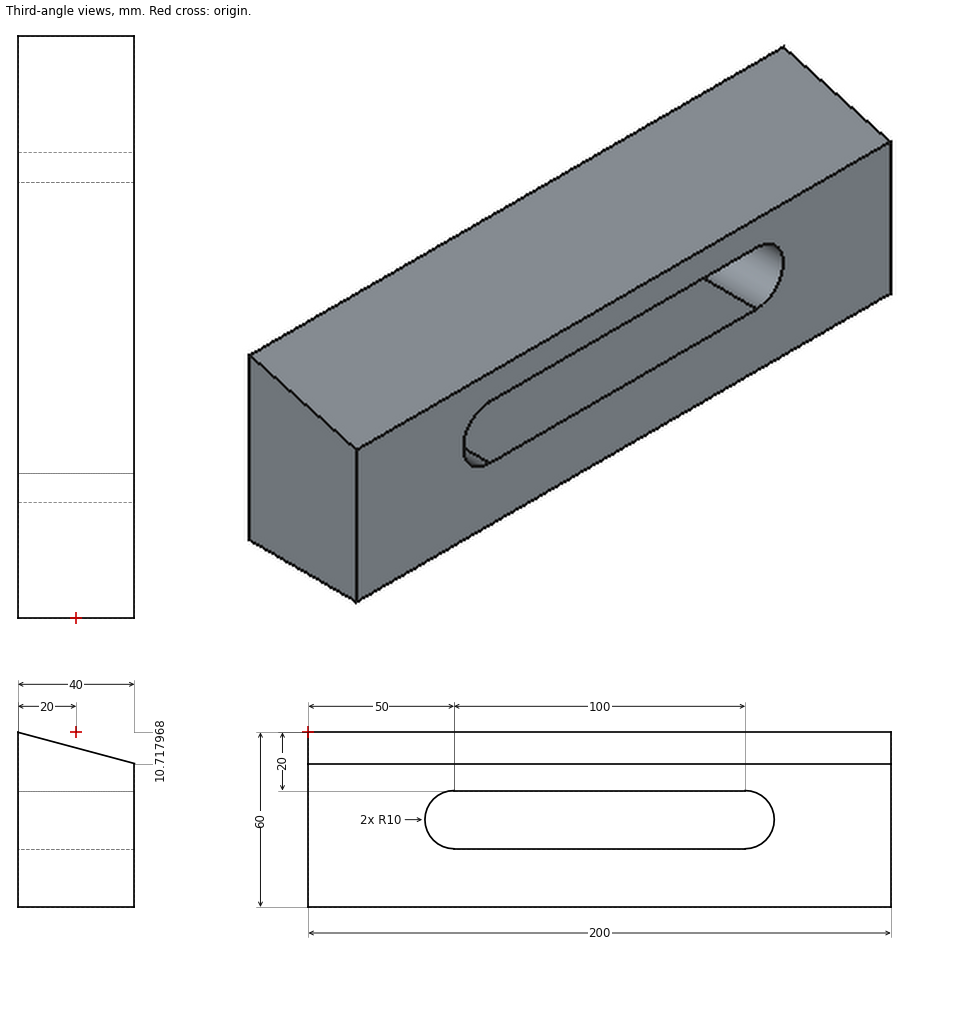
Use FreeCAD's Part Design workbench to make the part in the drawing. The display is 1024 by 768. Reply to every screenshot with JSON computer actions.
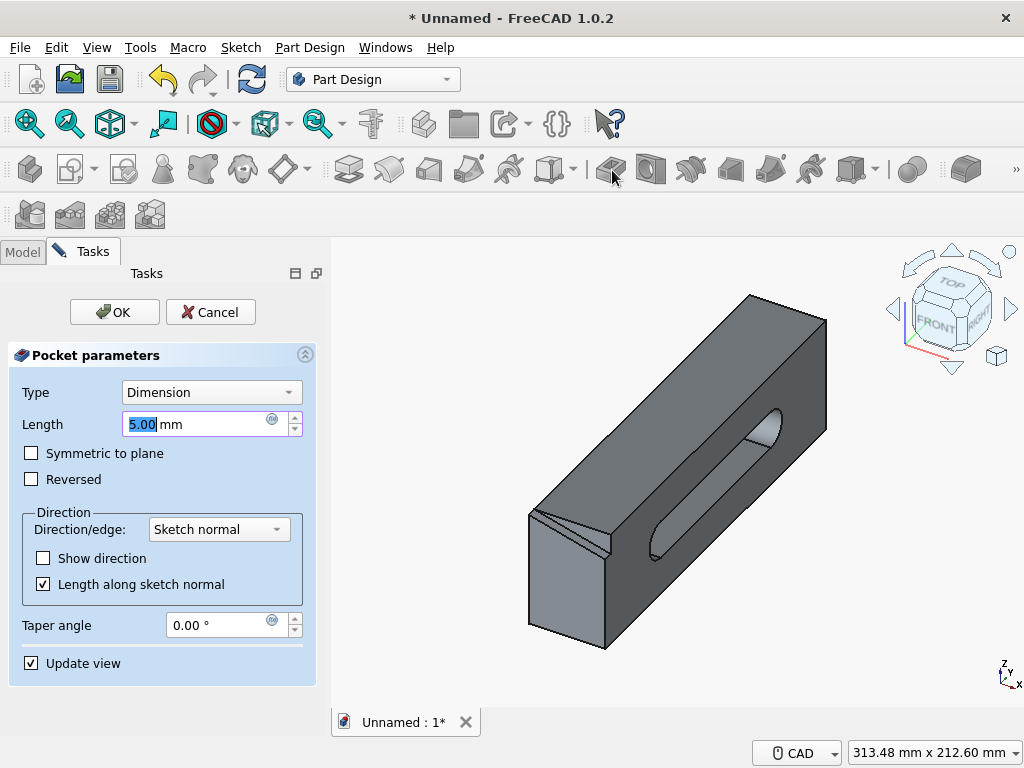
{"action": "left_click", "coordinate": [212, 392]}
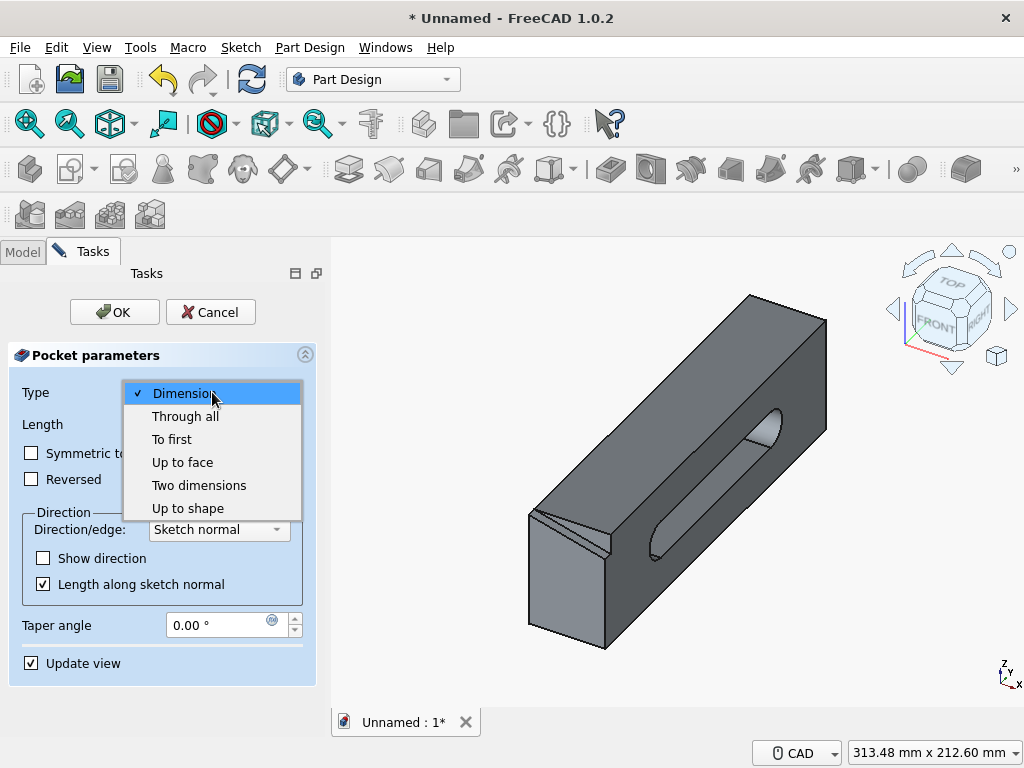
{"action": "left_click", "coordinate": [212, 416]}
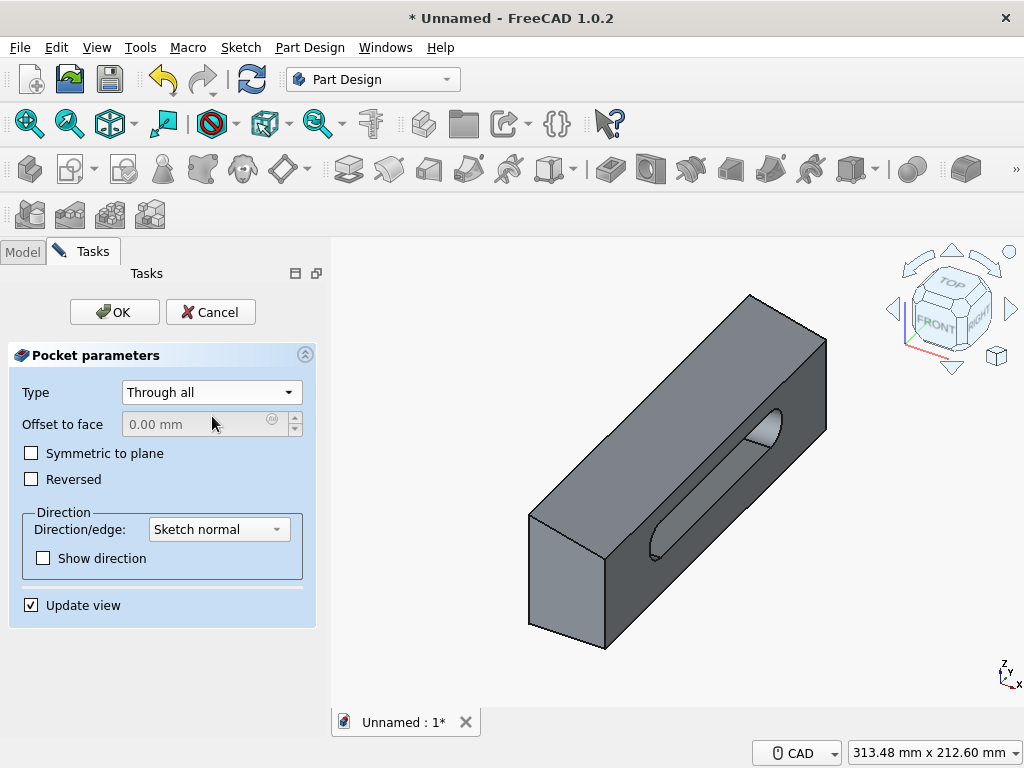
{"action": "left_click", "coordinate": [115, 312]}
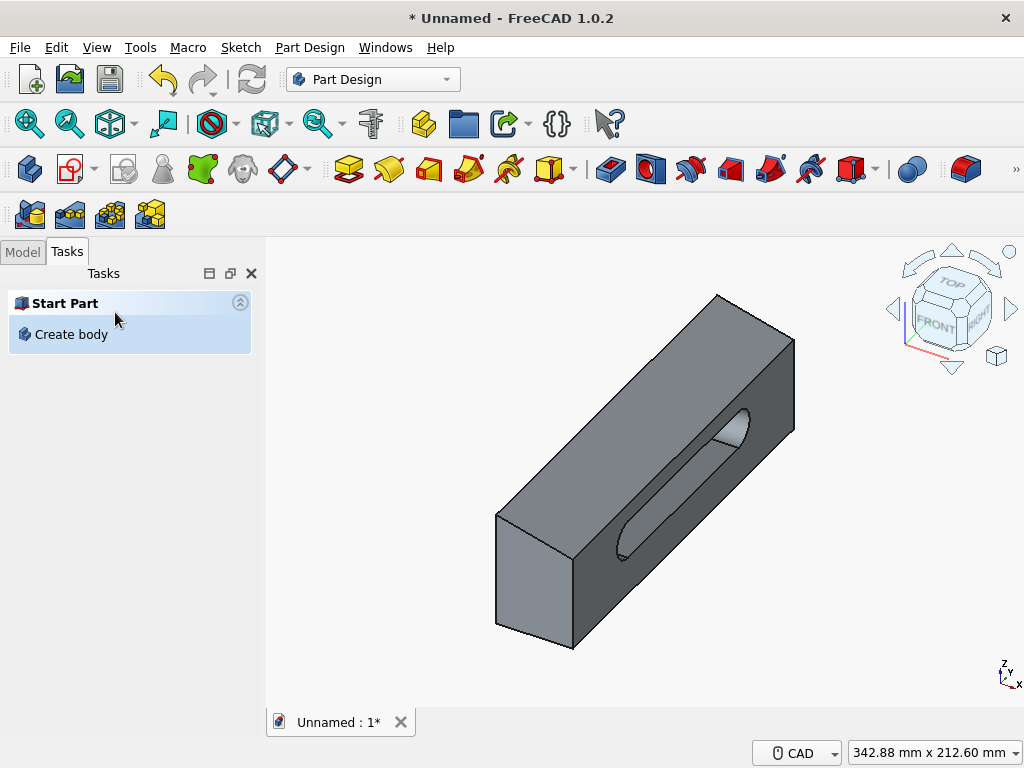
{"action": "key", "text": "0"}